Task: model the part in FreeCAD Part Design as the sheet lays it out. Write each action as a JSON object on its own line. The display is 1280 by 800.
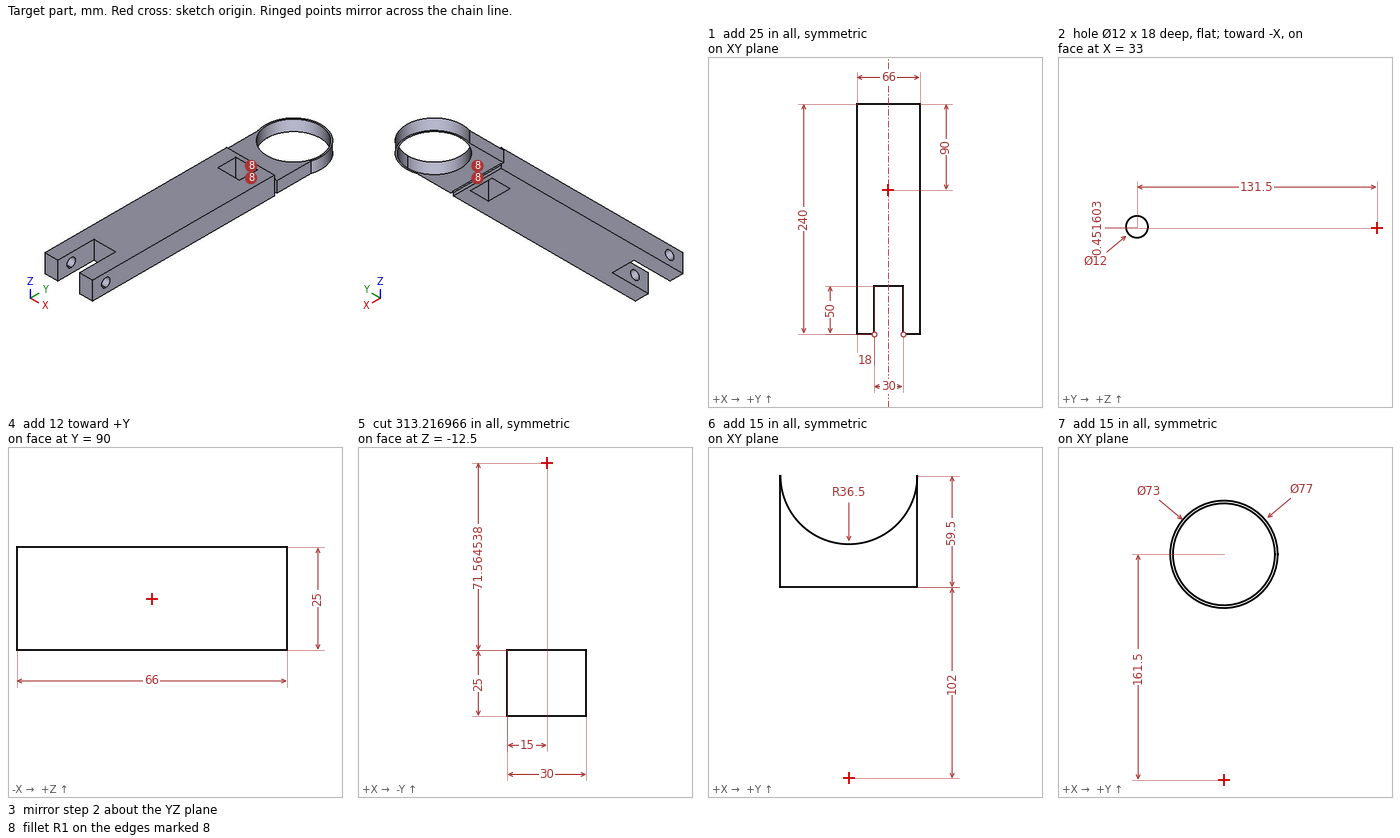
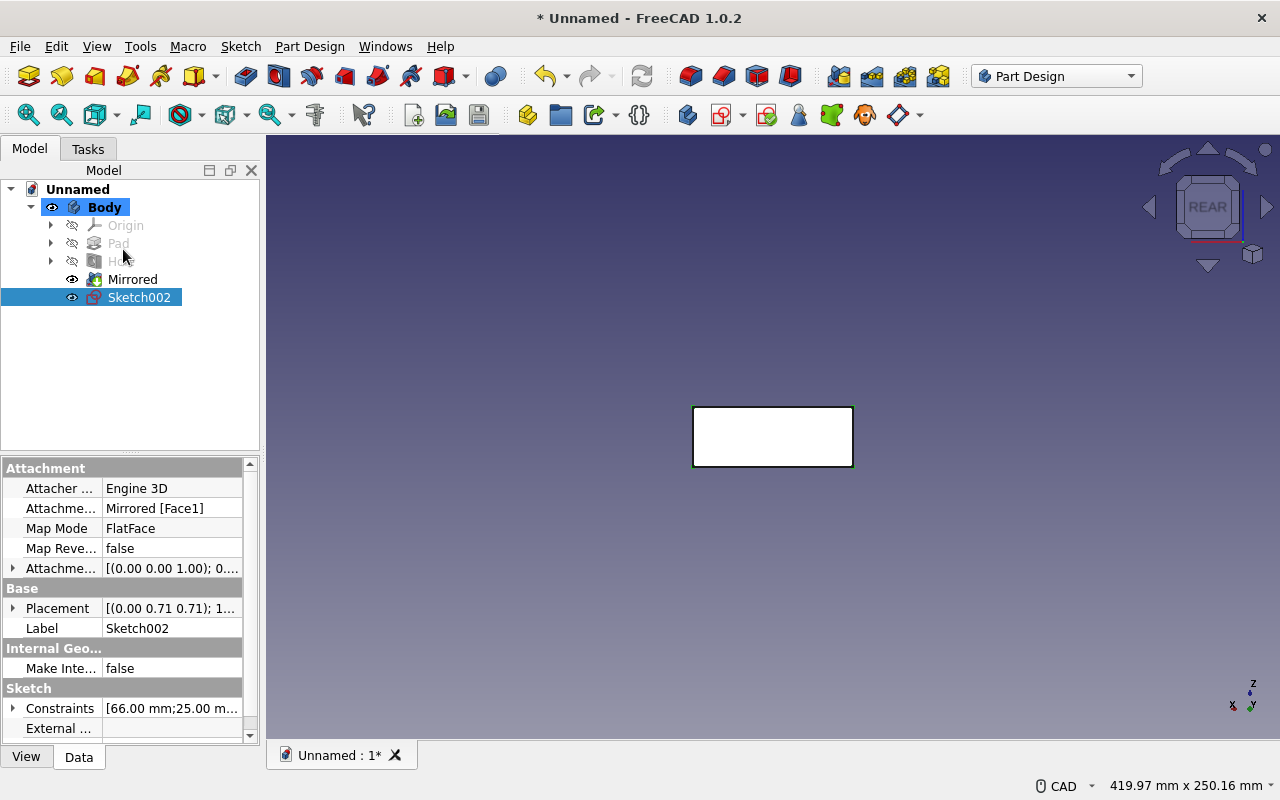
{"action": "left_click", "coordinate": [29, 76]}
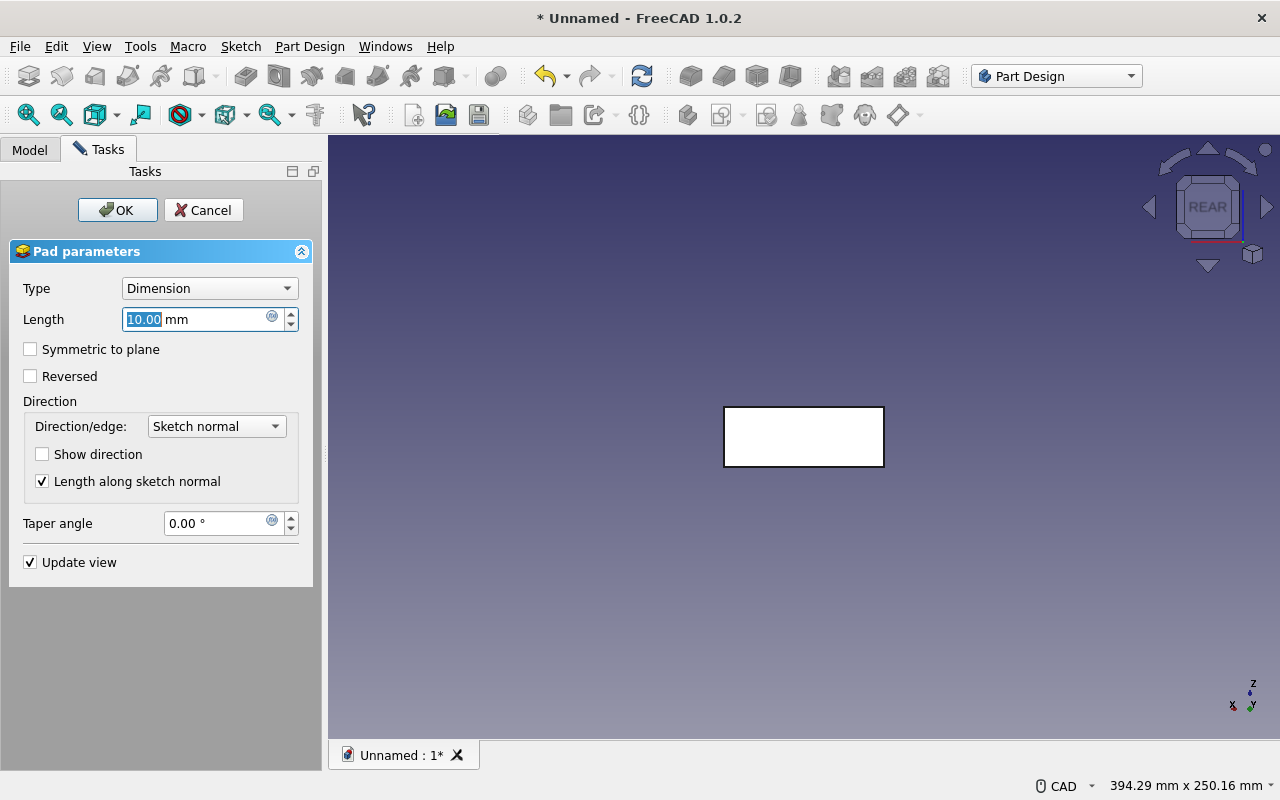
{"action": "type", "text": "12"}
{"action": "key", "text": "Tab"}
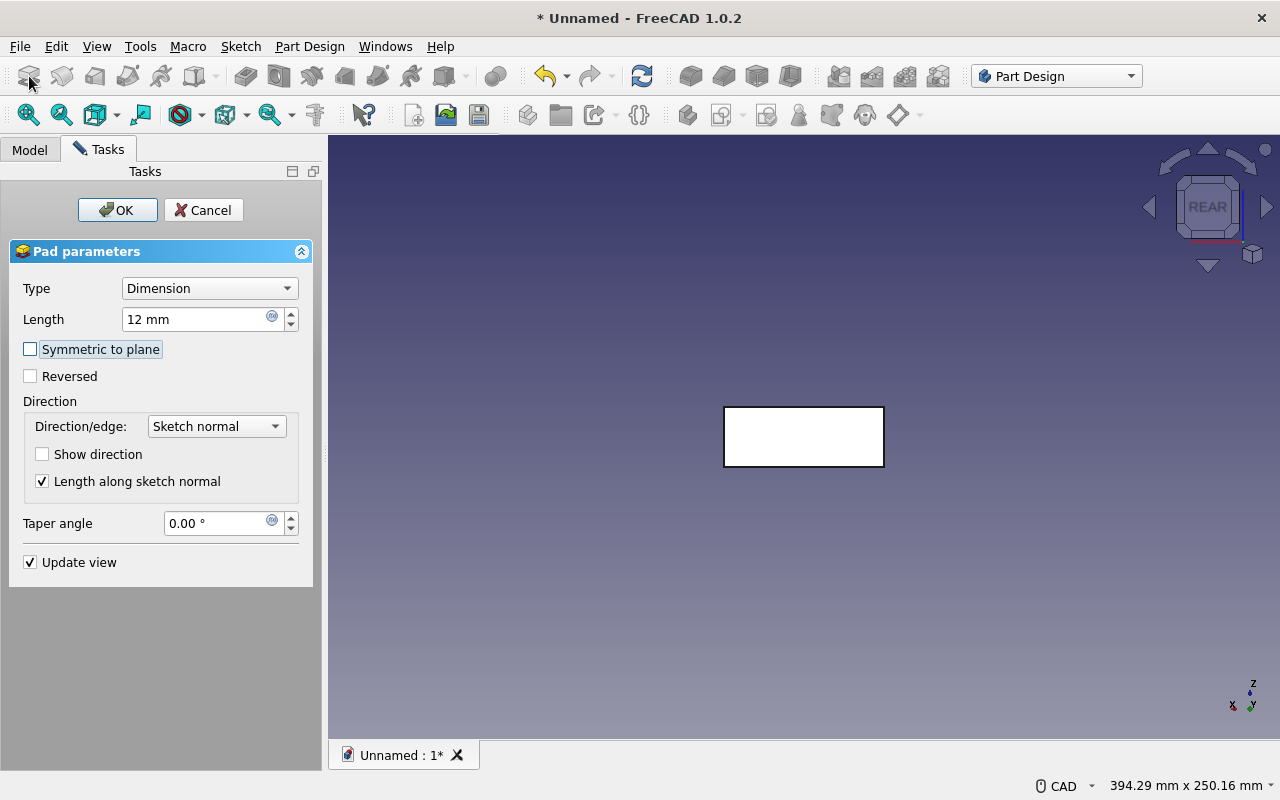
{"action": "left_click", "coordinate": [118, 210]}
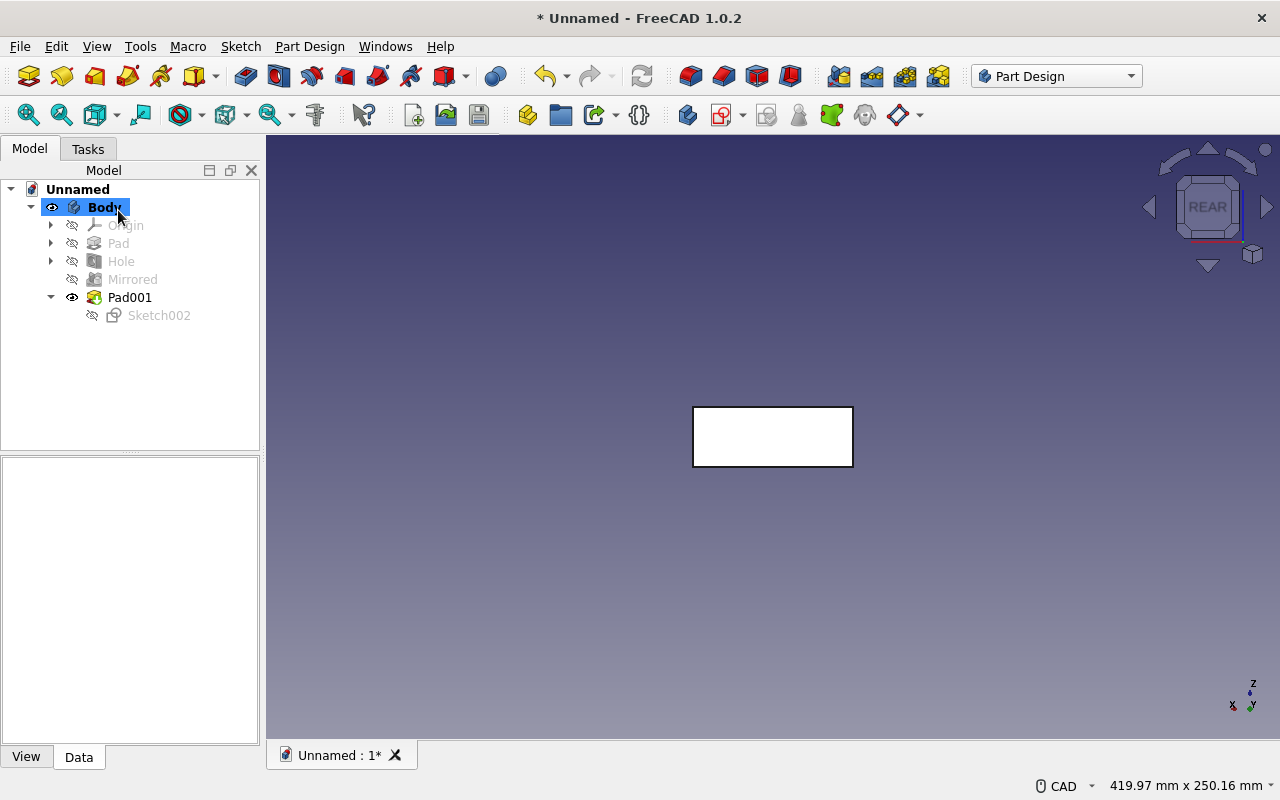
{"action": "key", "text": "v f"}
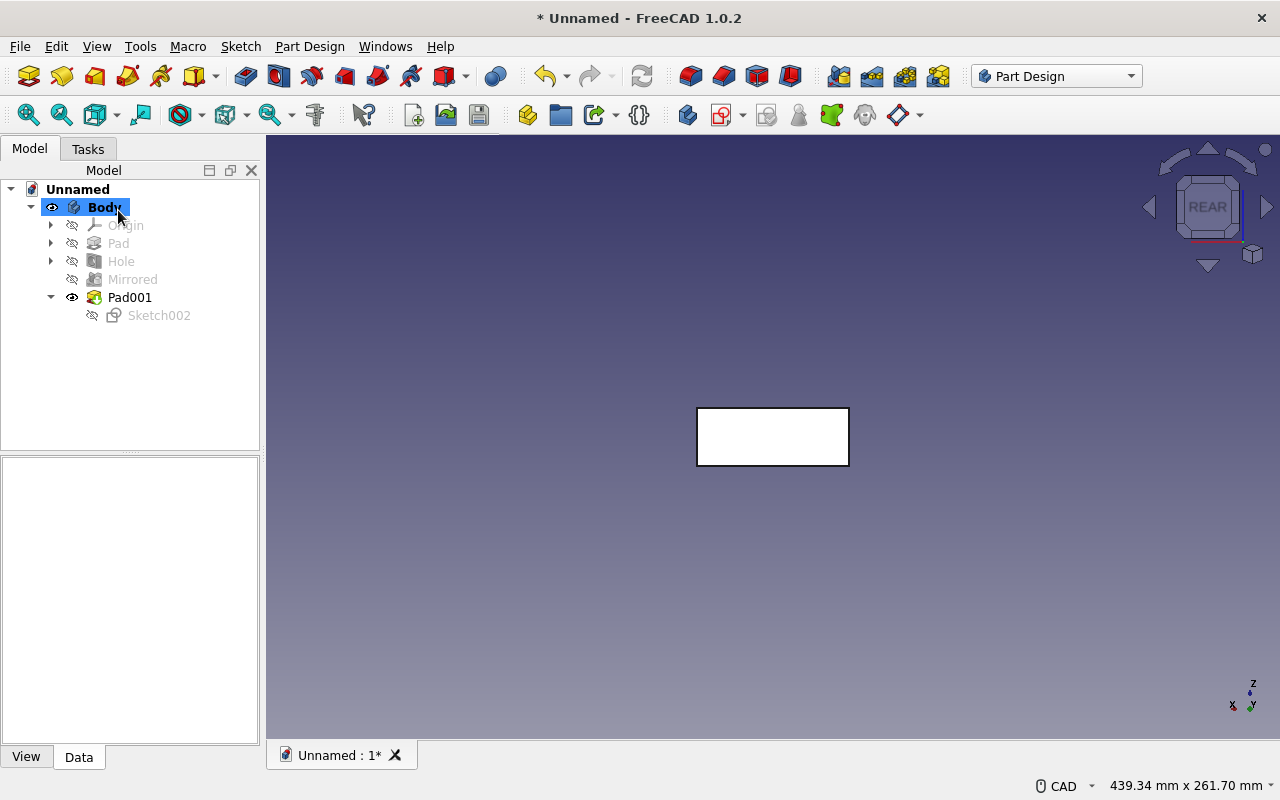
{"action": "key", "text": "5"}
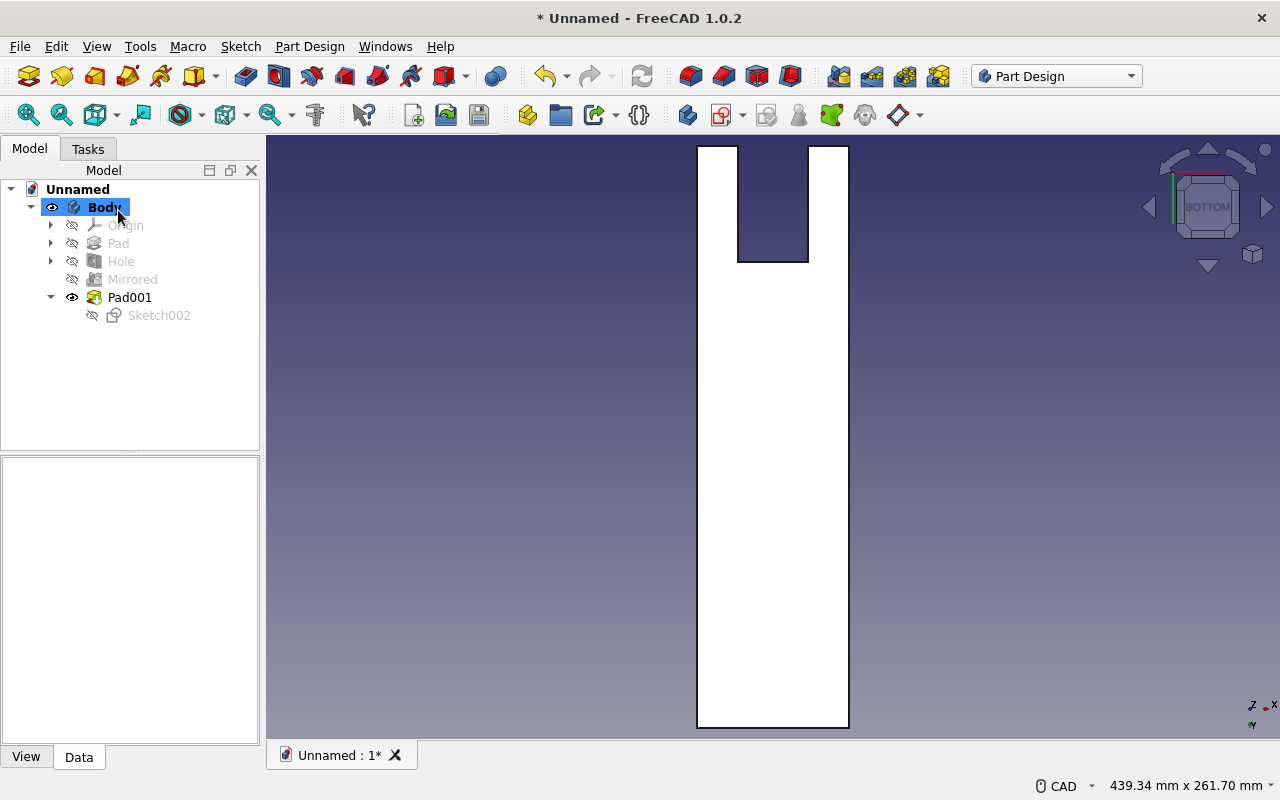
{"action": "left_click", "coordinate": [773, 602]}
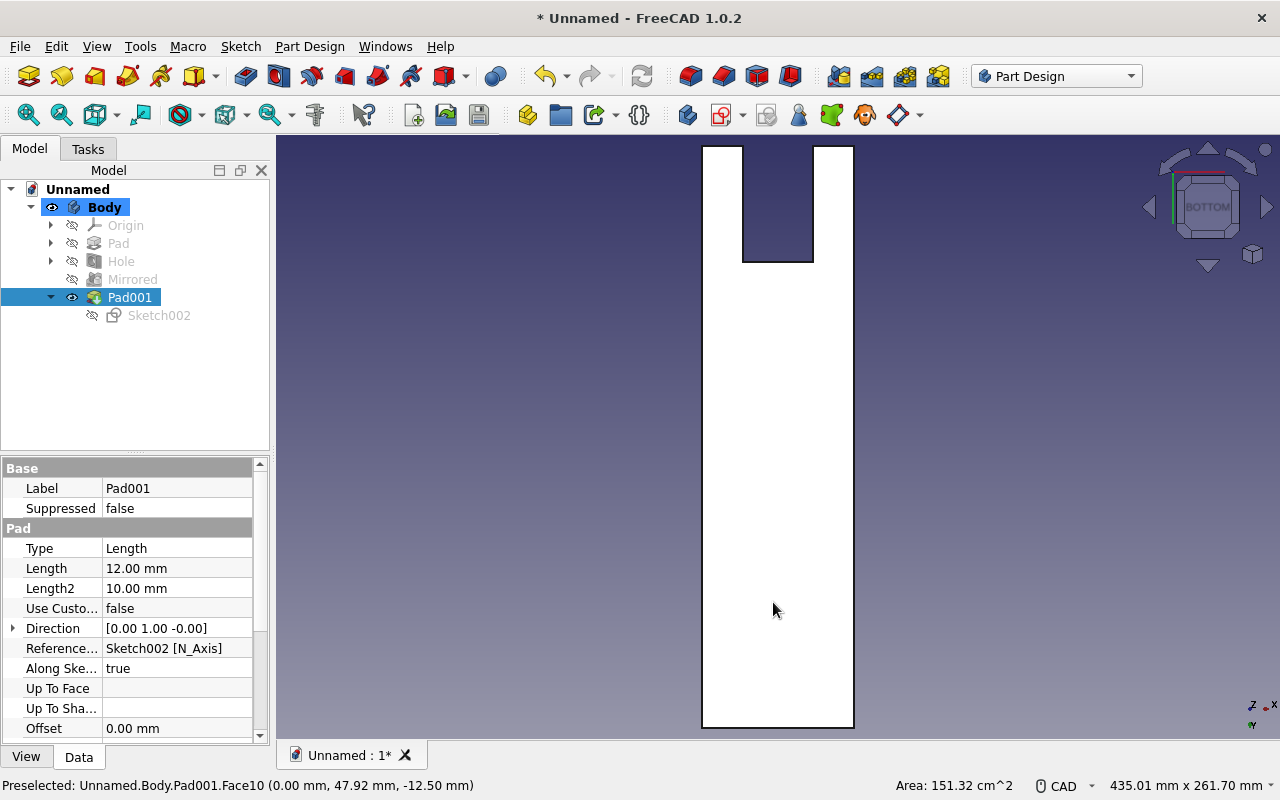
{"action": "left_click", "coordinate": [720, 116]}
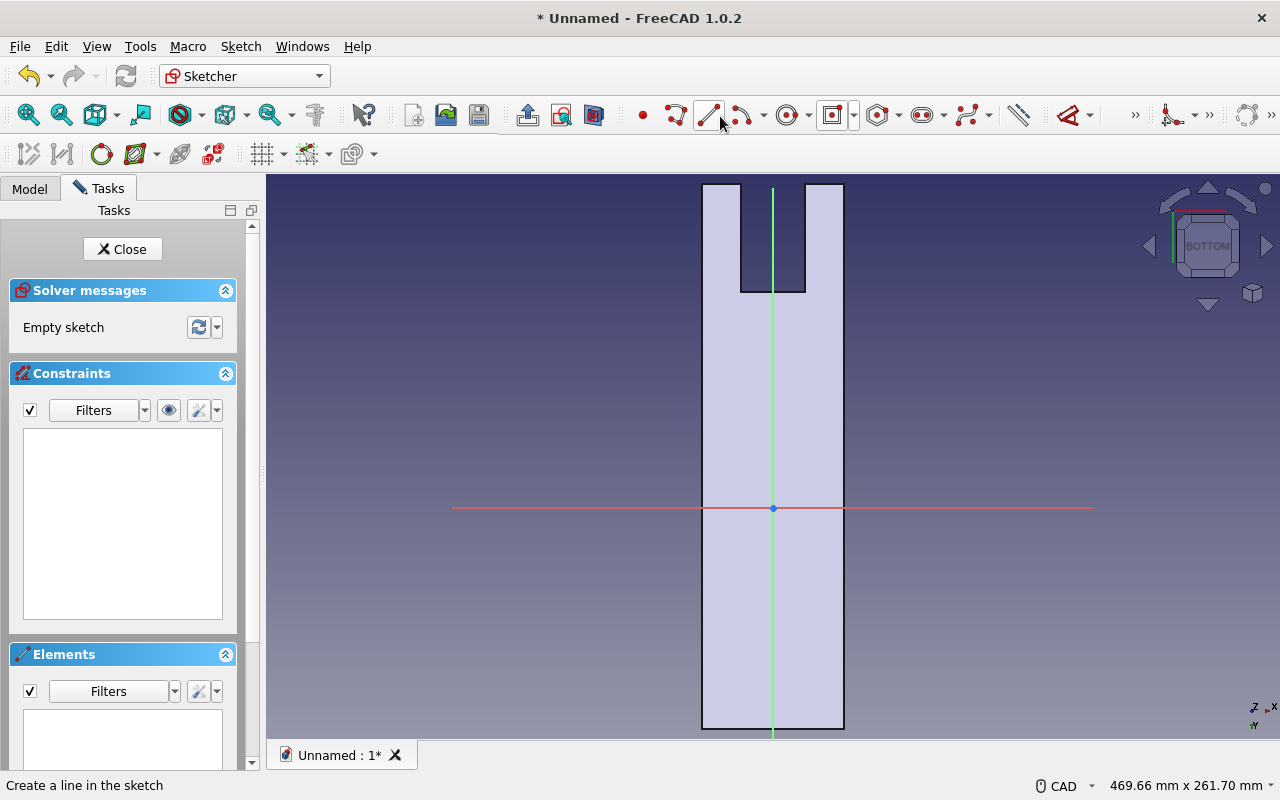
{"action": "scroll", "coordinate": [704, 456], "scroll_direction": "down", "scroll_amount": 5}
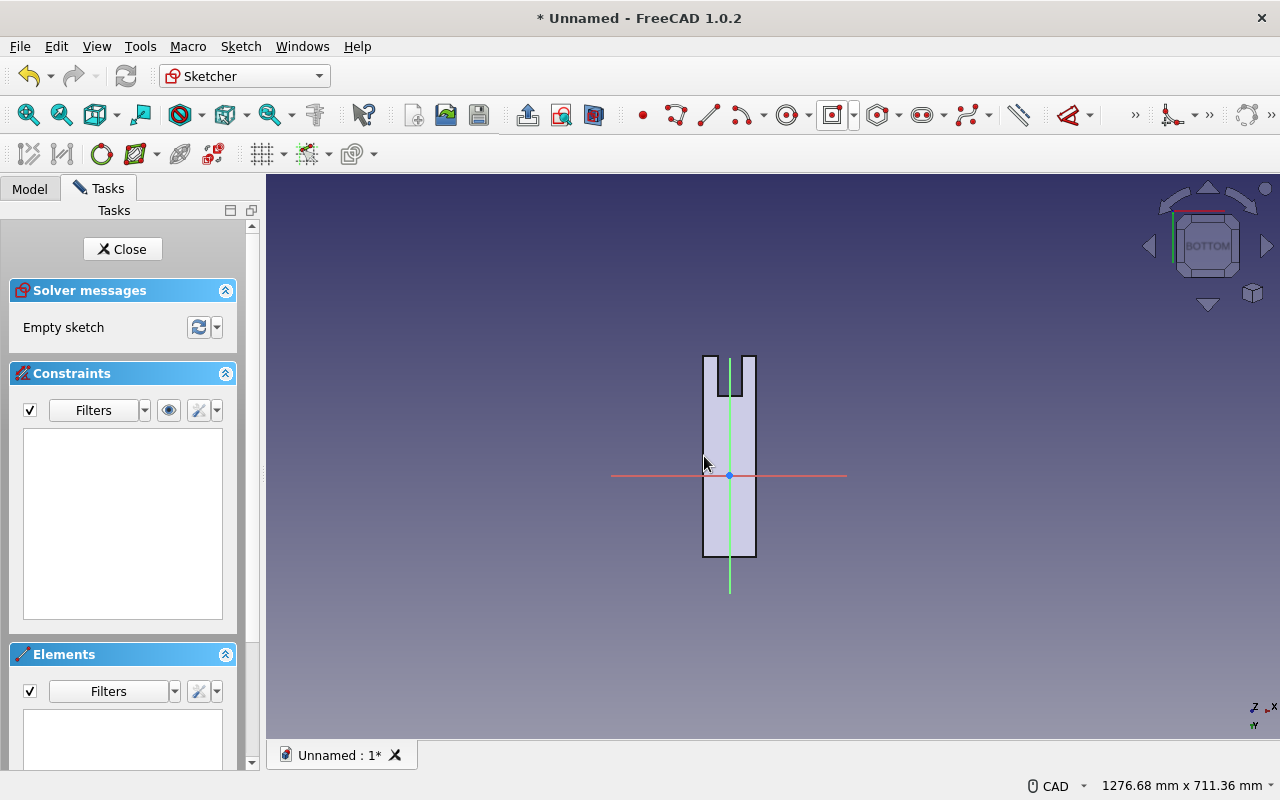
{"action": "scroll", "coordinate": [731, 548], "scroll_direction": "up", "scroll_amount": 14}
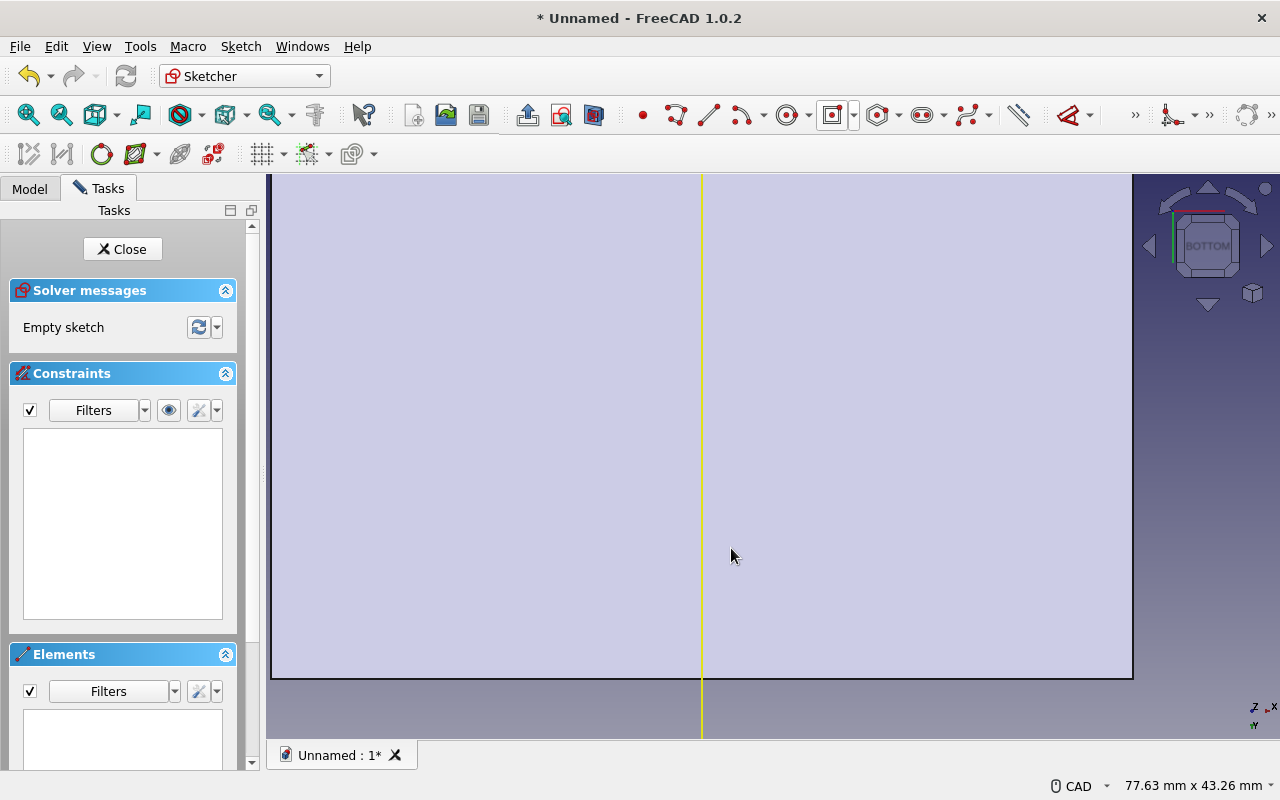
{"action": "key", "text": "g r"}